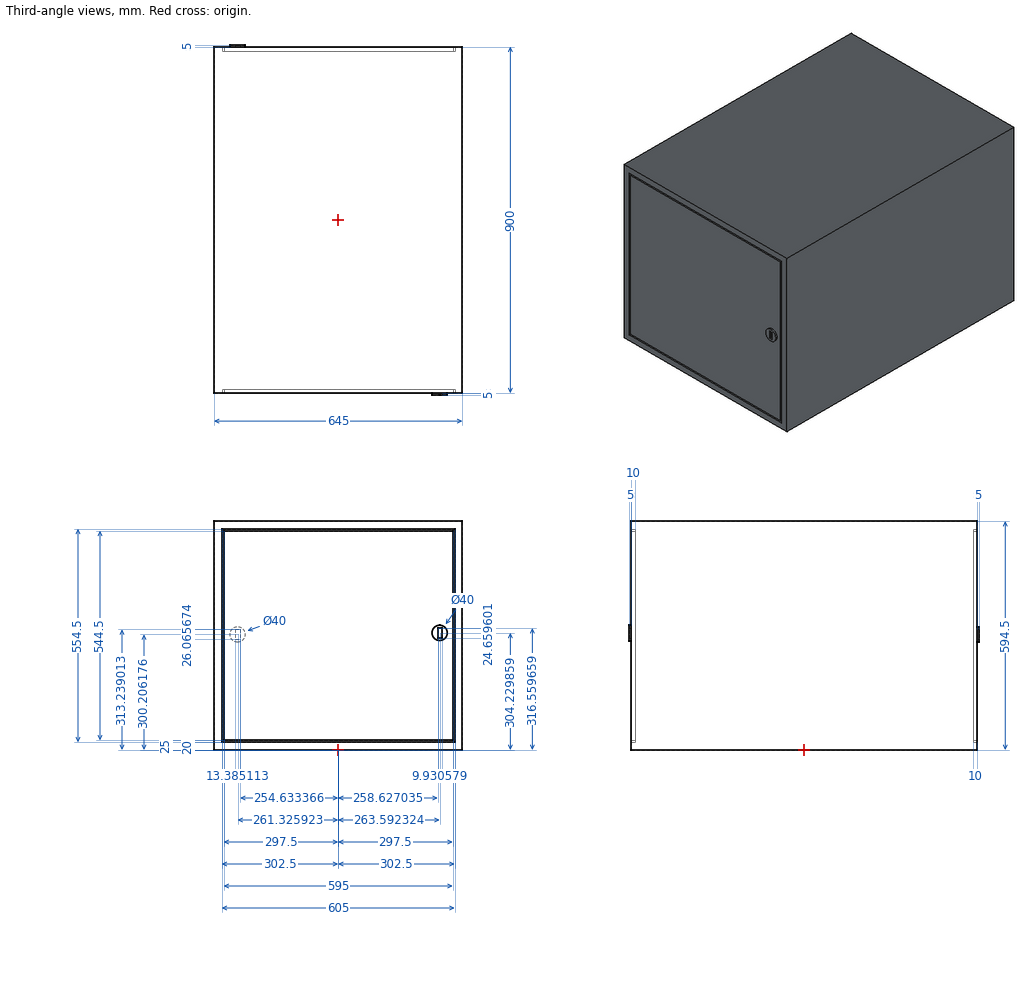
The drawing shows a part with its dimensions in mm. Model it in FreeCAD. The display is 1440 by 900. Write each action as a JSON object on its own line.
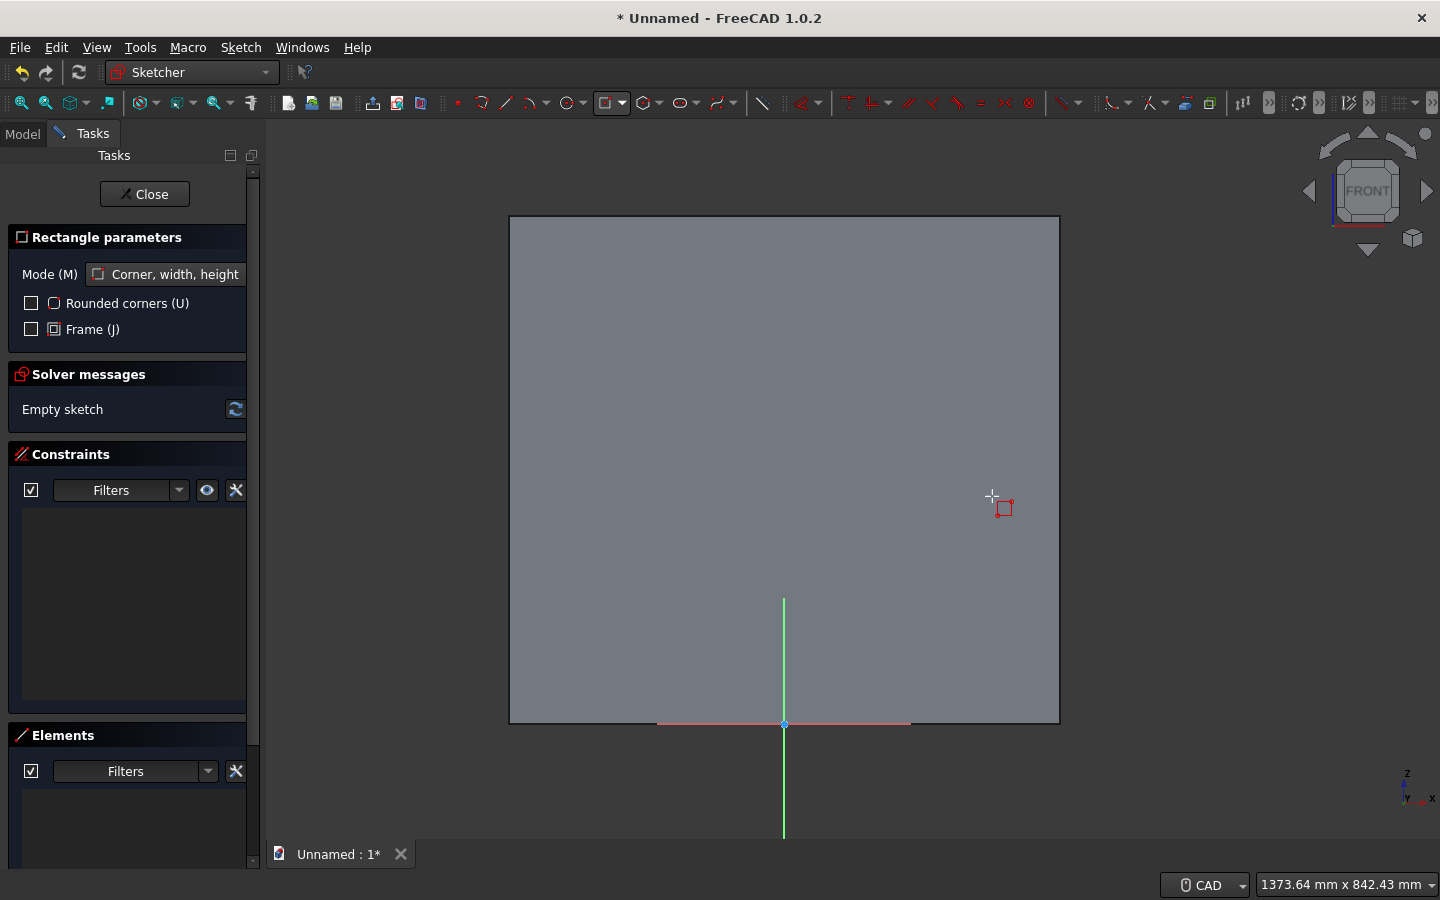
{"action": "left_click", "coordinate": [526, 233]}
{"action": "left_click", "coordinate": [1043, 707]}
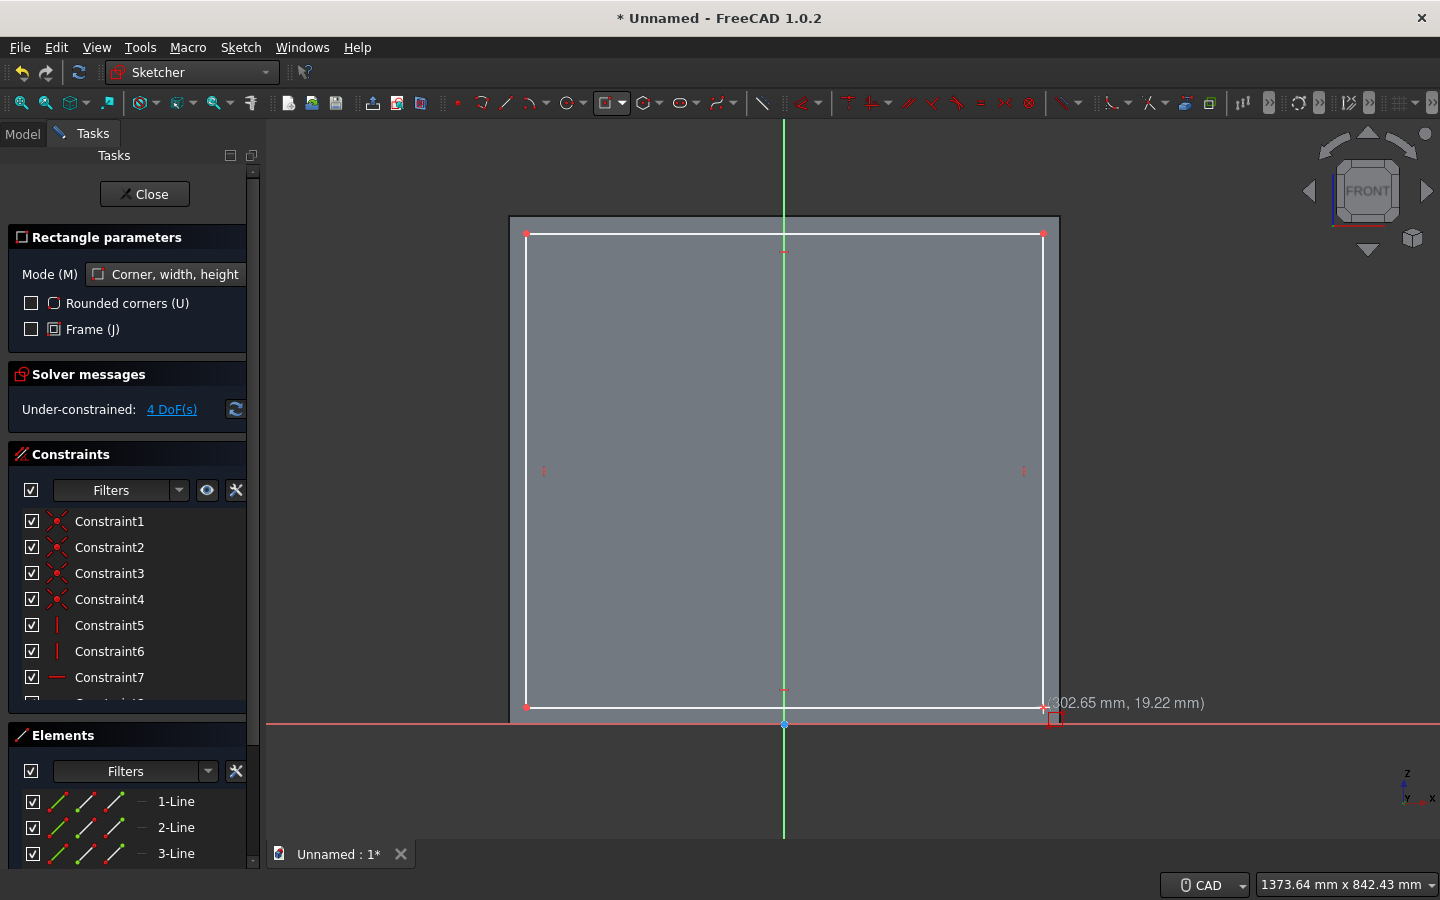
{"action": "scroll", "coordinate": [530, 238], "scroll_direction": "up", "scroll_amount": 7}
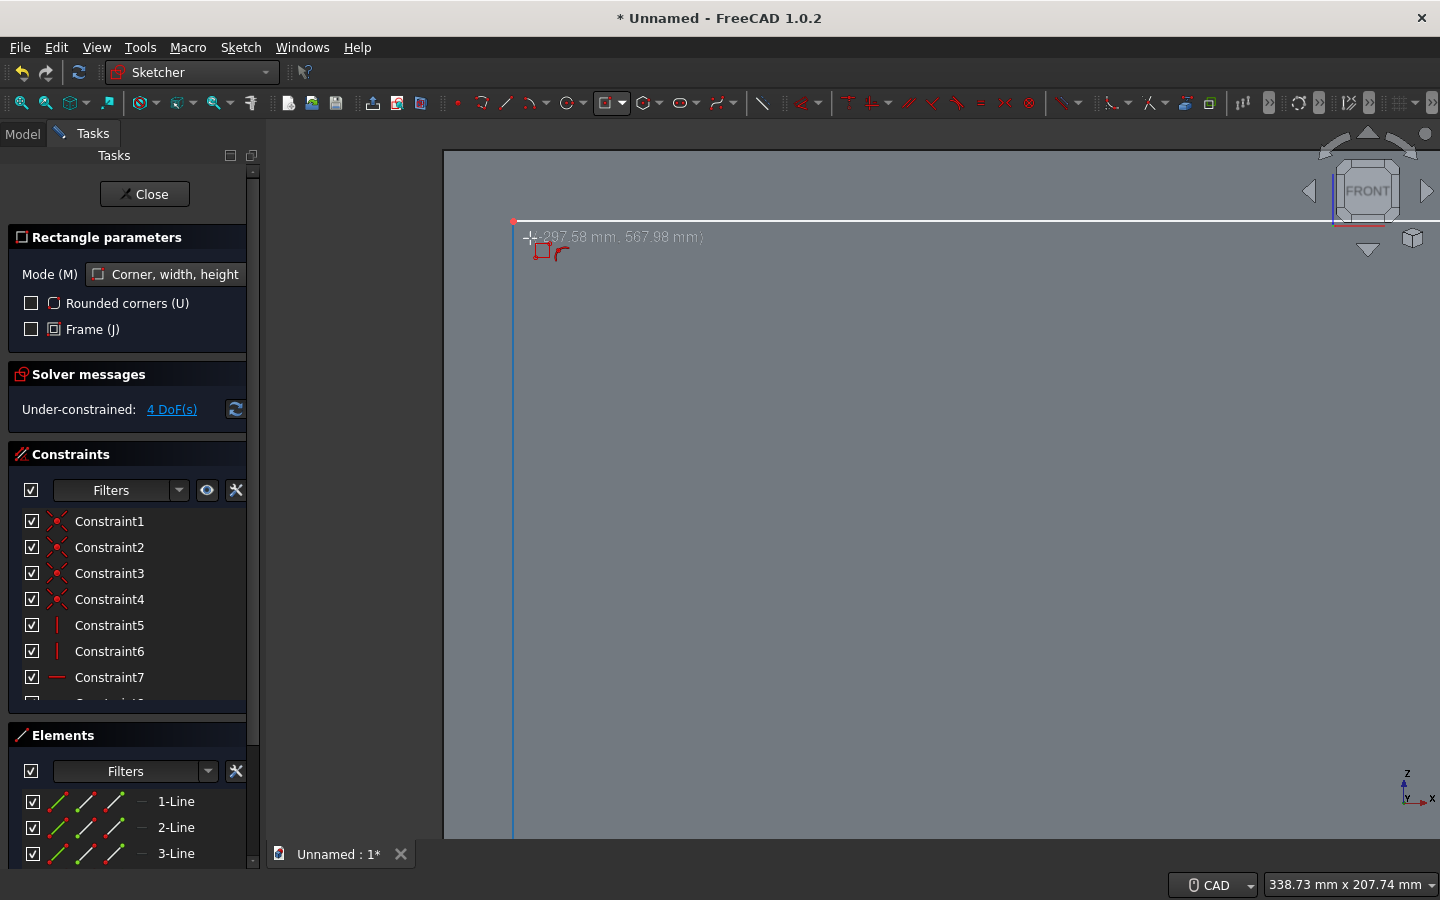
{"action": "left_click", "coordinate": [530, 236]}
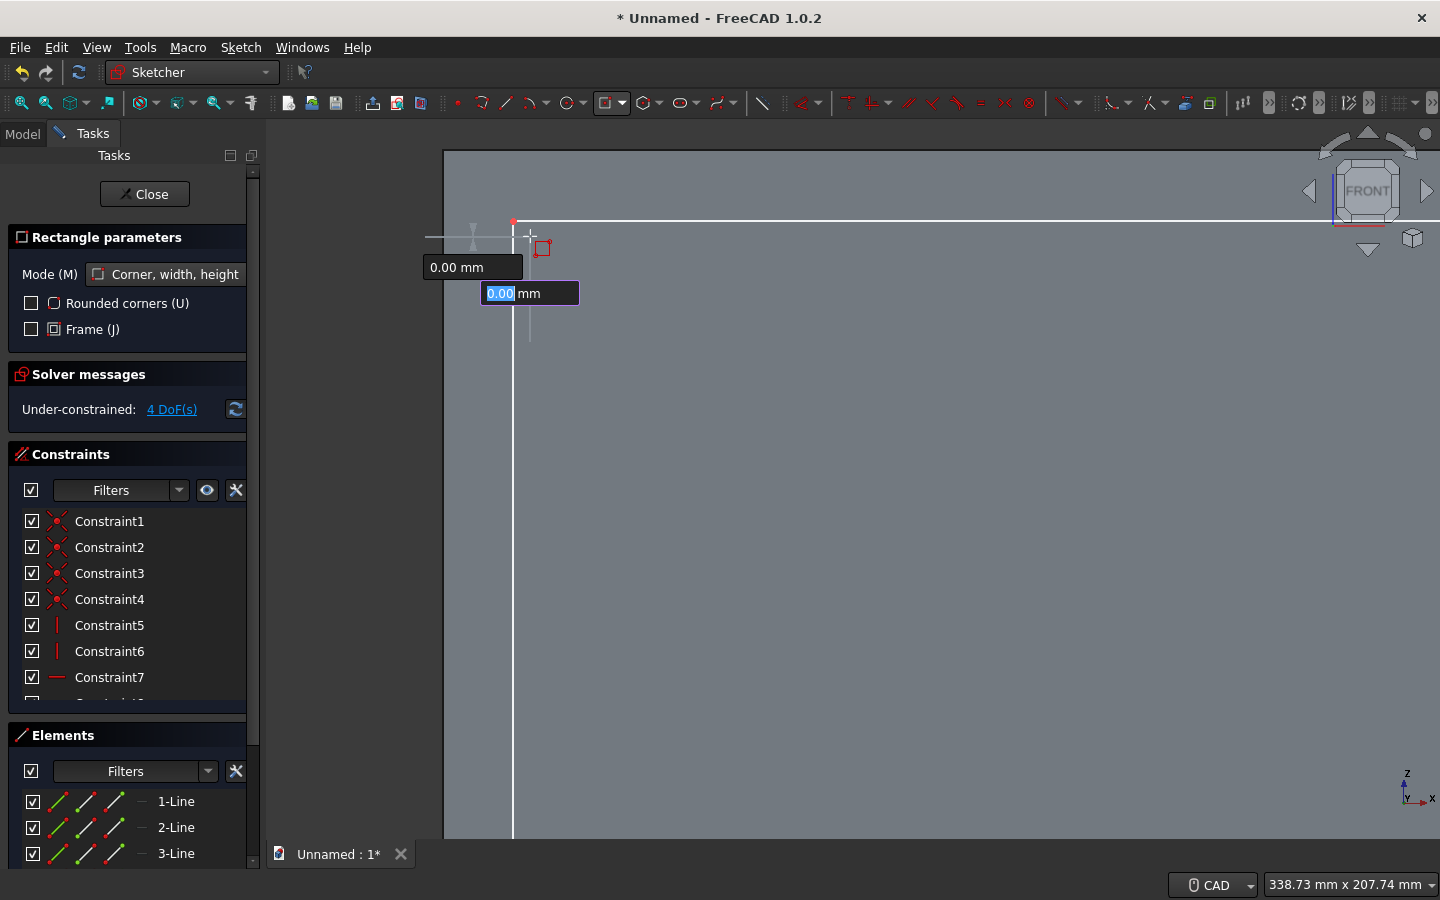
{"action": "scroll", "coordinate": [530, 238], "scroll_direction": "down", "scroll_amount": 7}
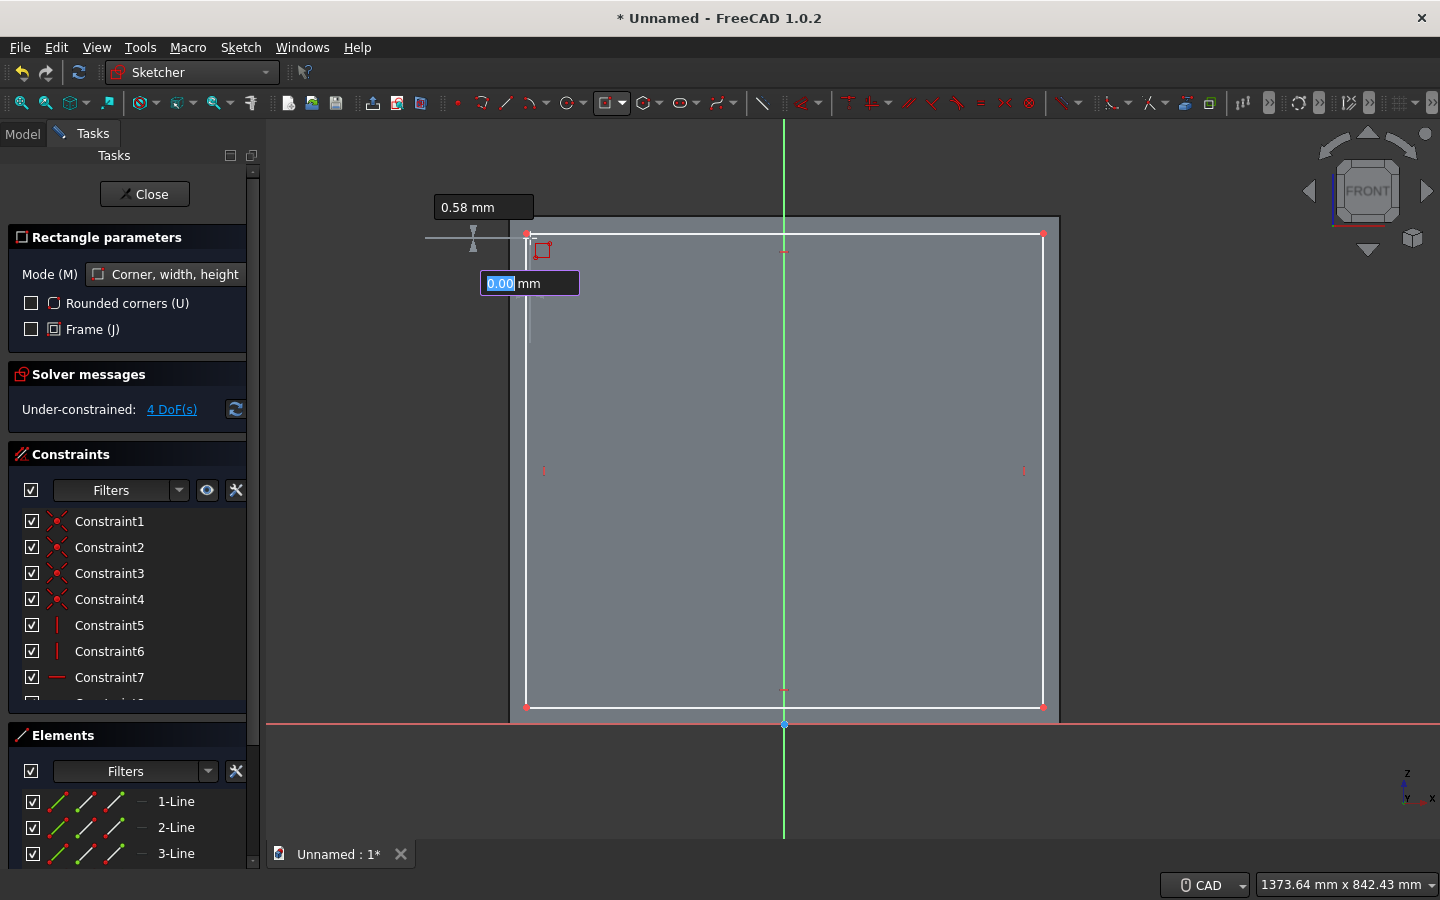
{"action": "scroll", "coordinate": [1039, 703], "scroll_direction": "up", "scroll_amount": 7}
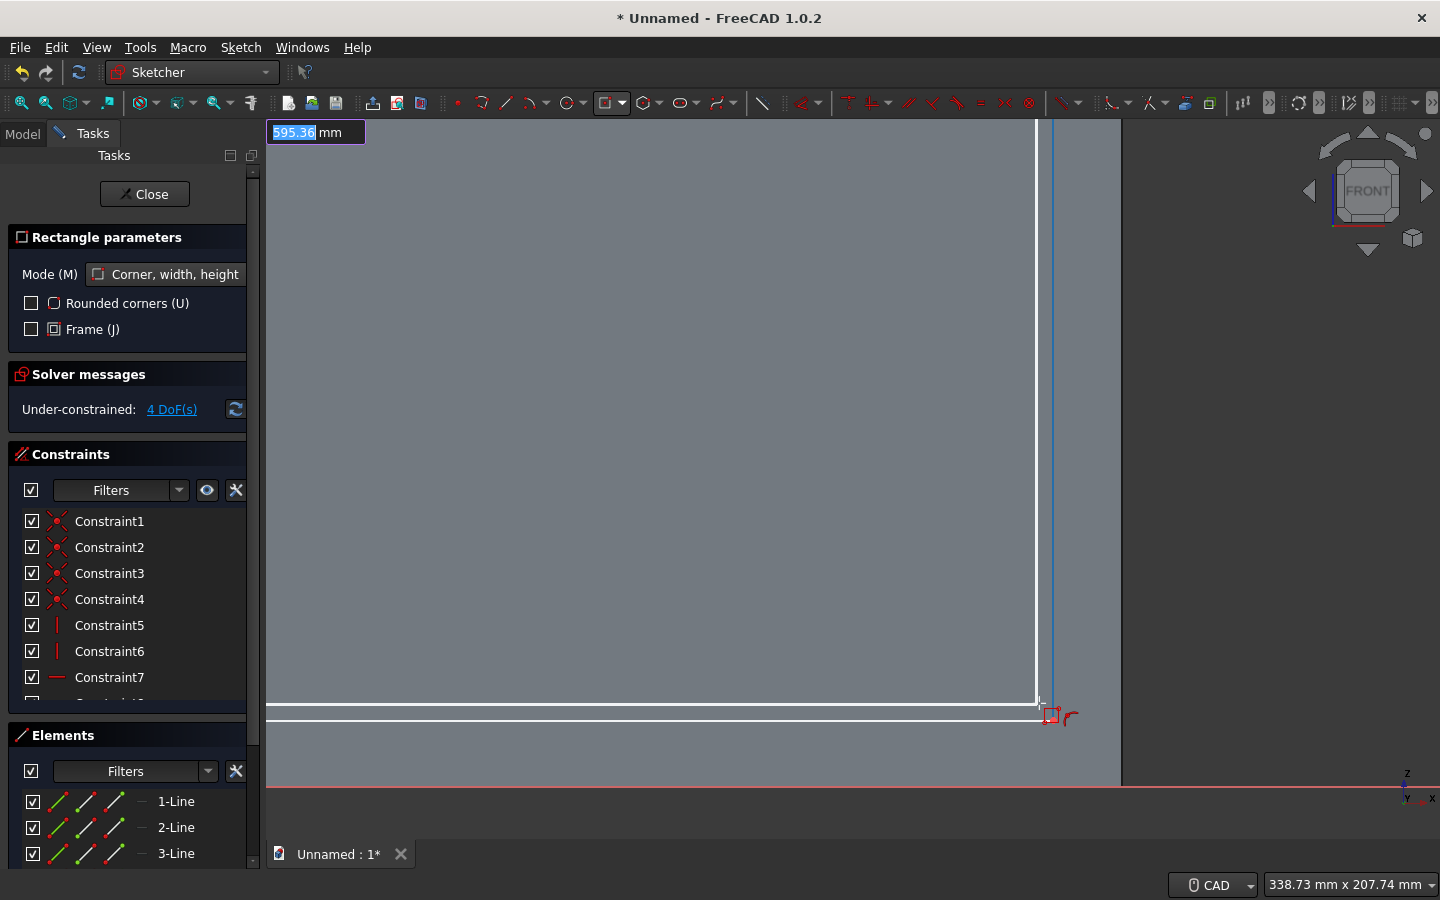
{"action": "left_click", "coordinate": [1035, 701]}
{"action": "key", "text": "Escape"}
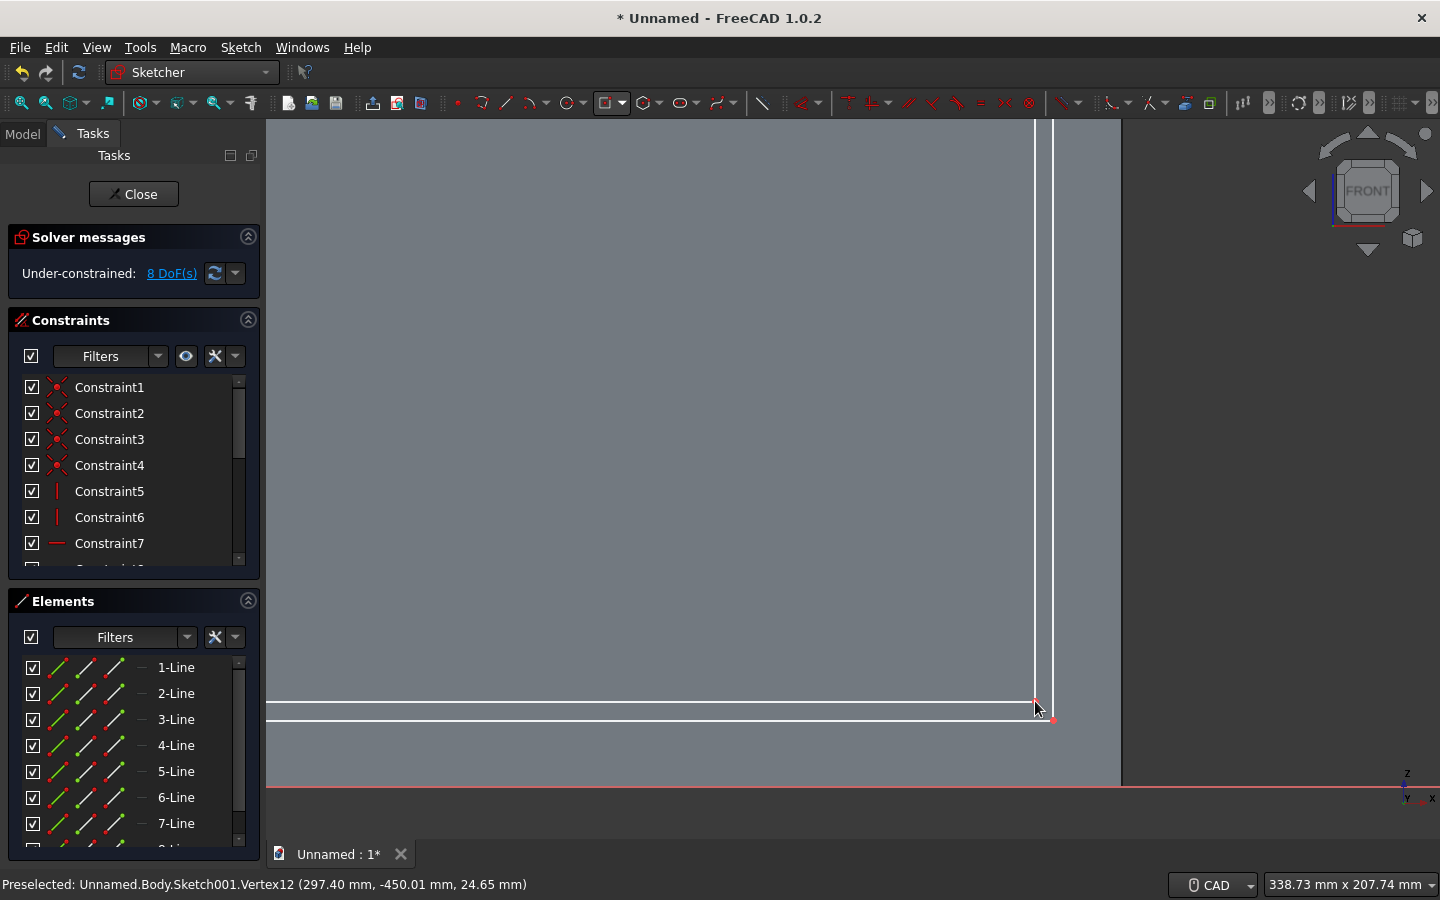
{"action": "key", "text": "d"}